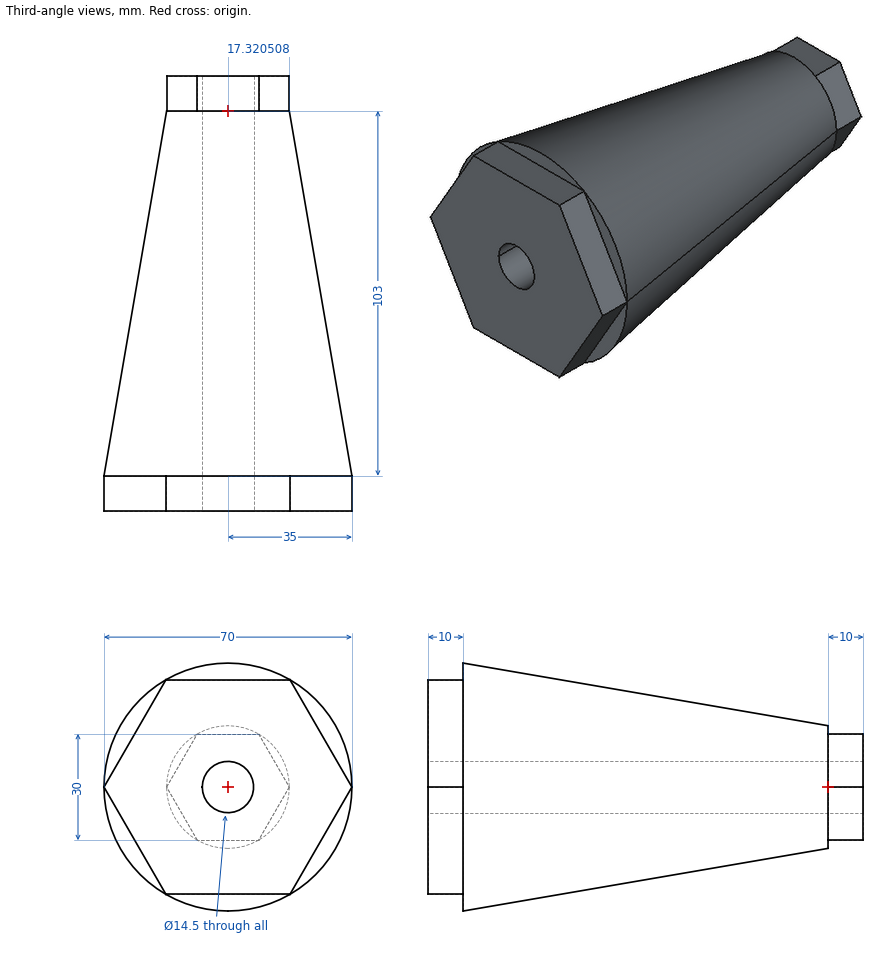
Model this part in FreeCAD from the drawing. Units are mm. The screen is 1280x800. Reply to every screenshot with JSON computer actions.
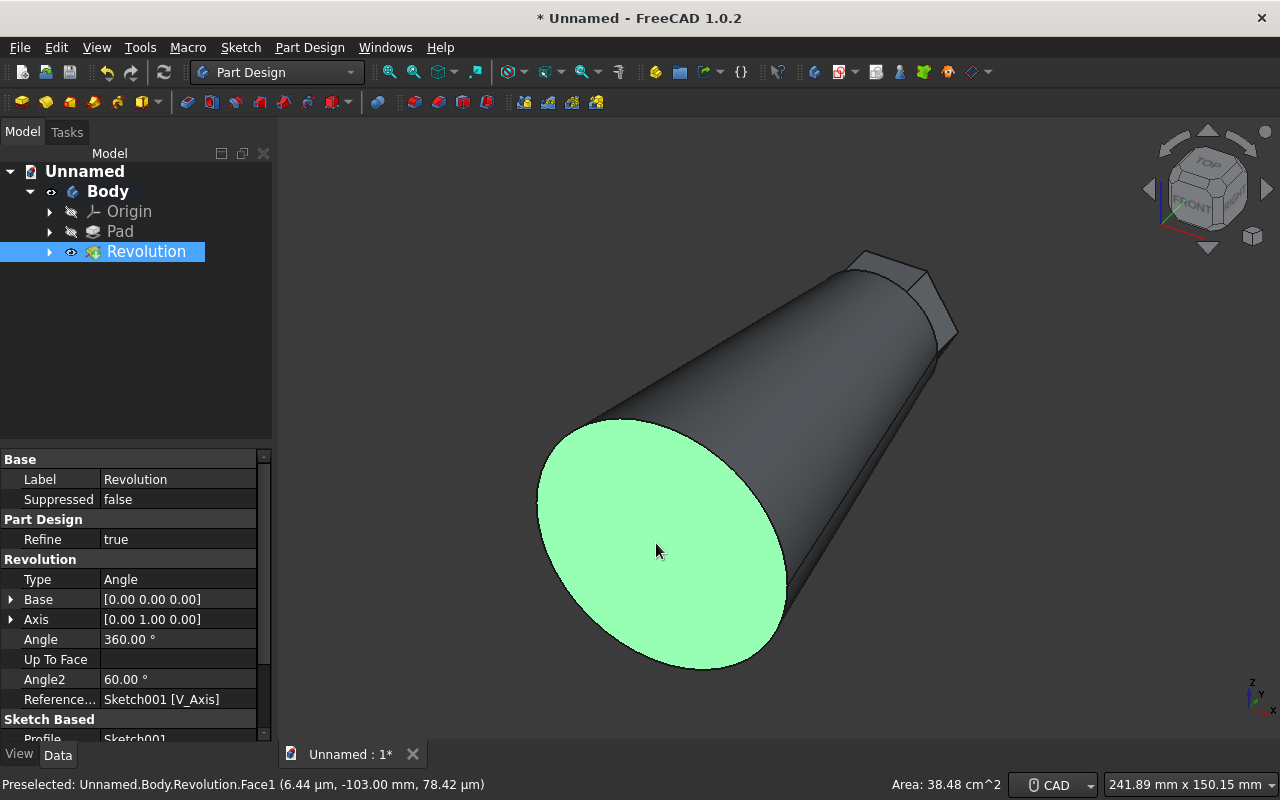
{"action": "left_click", "coordinate": [840, 72]}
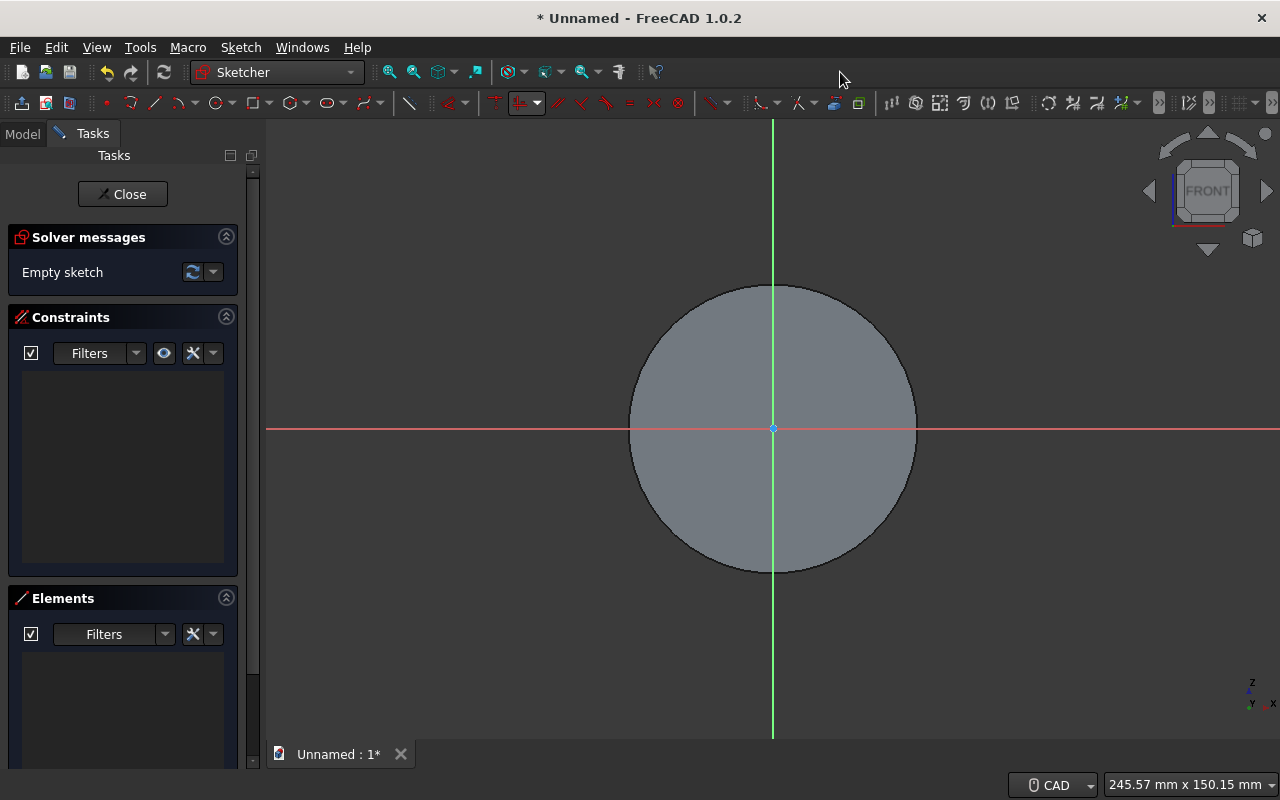
{"action": "scroll", "coordinate": [912, 429], "scroll_direction": "up", "scroll_amount": 2}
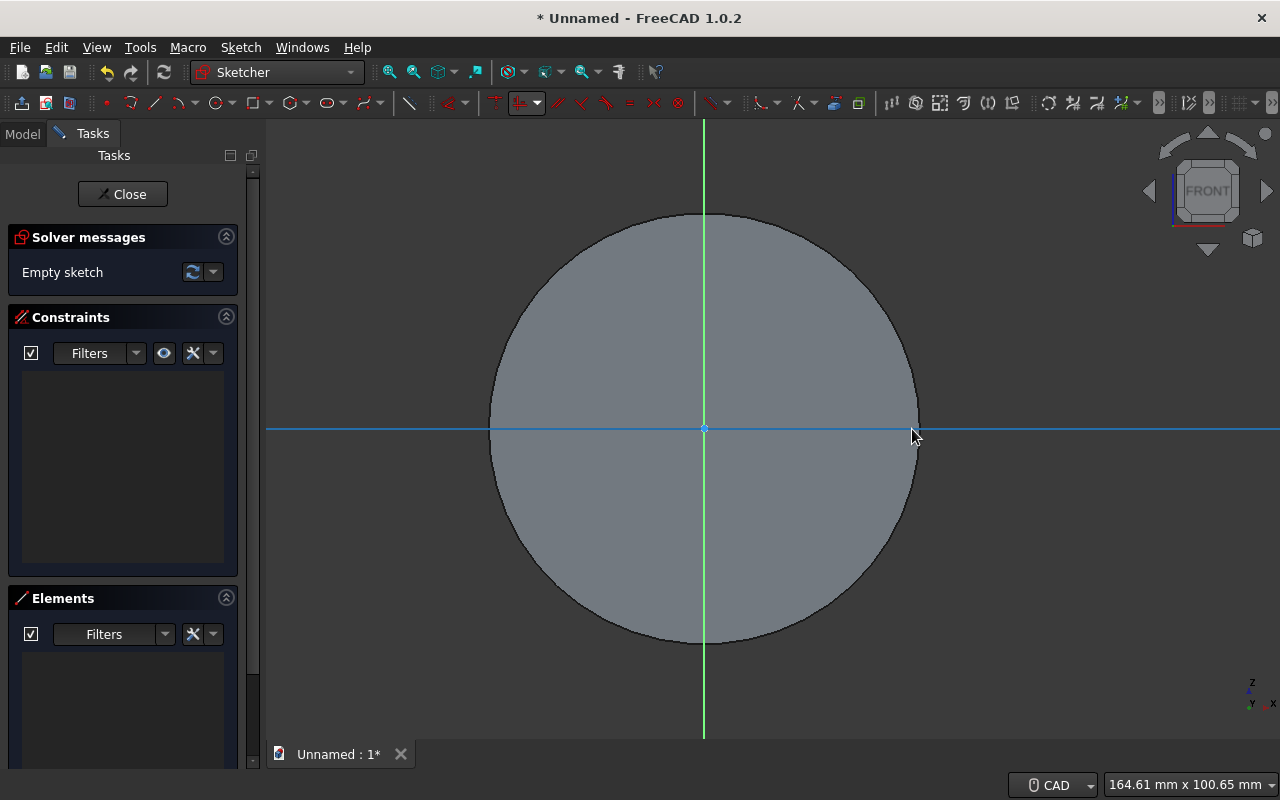
{"action": "left_click", "coordinate": [290, 104]}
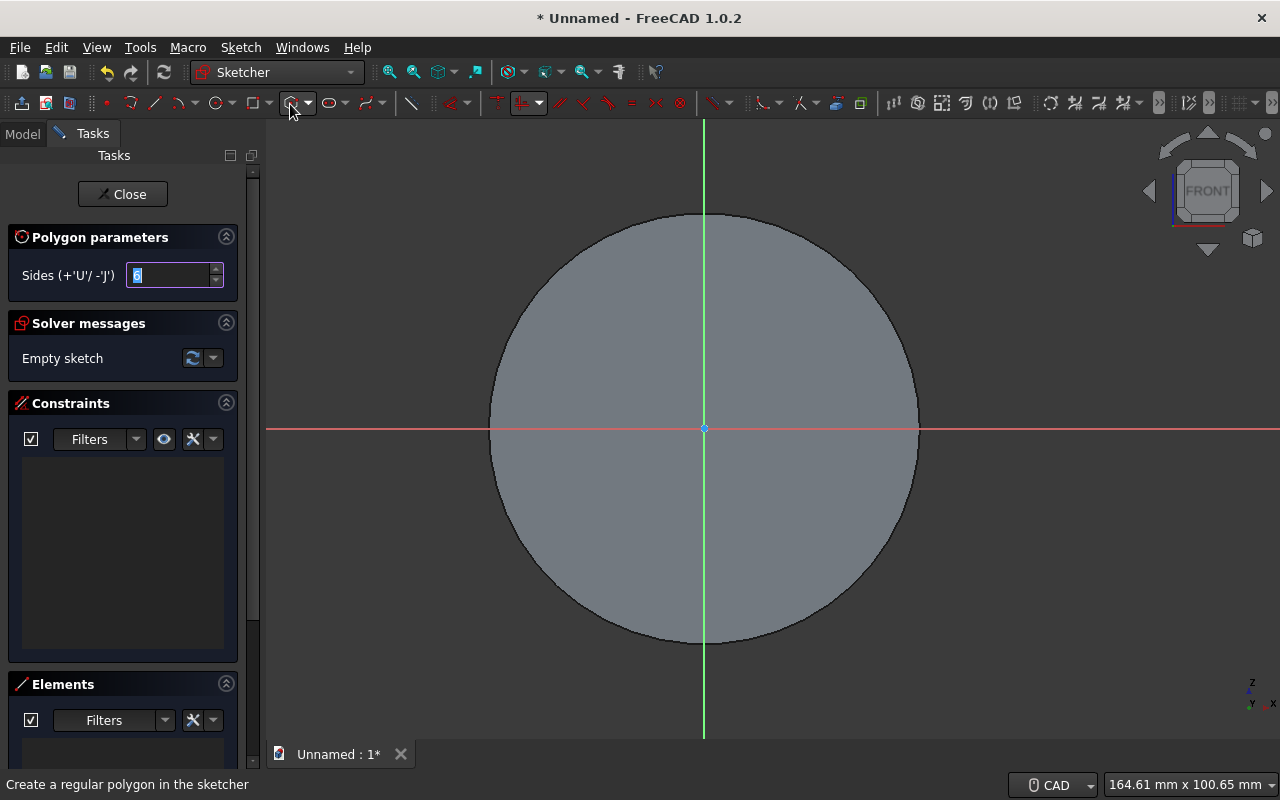
{"action": "left_click", "coordinate": [704, 429]}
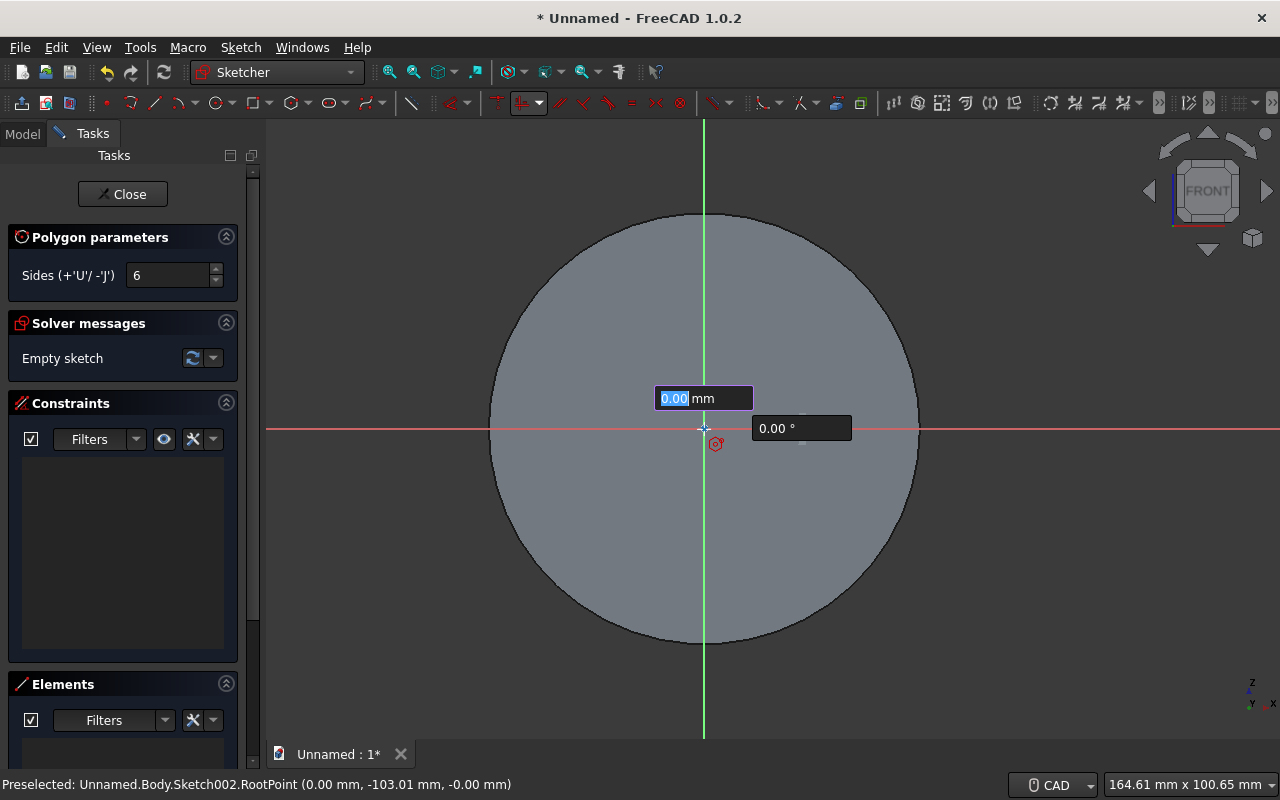
{"action": "left_click", "coordinate": [489, 429]}
{"action": "right_click", "coordinate": [489, 429]}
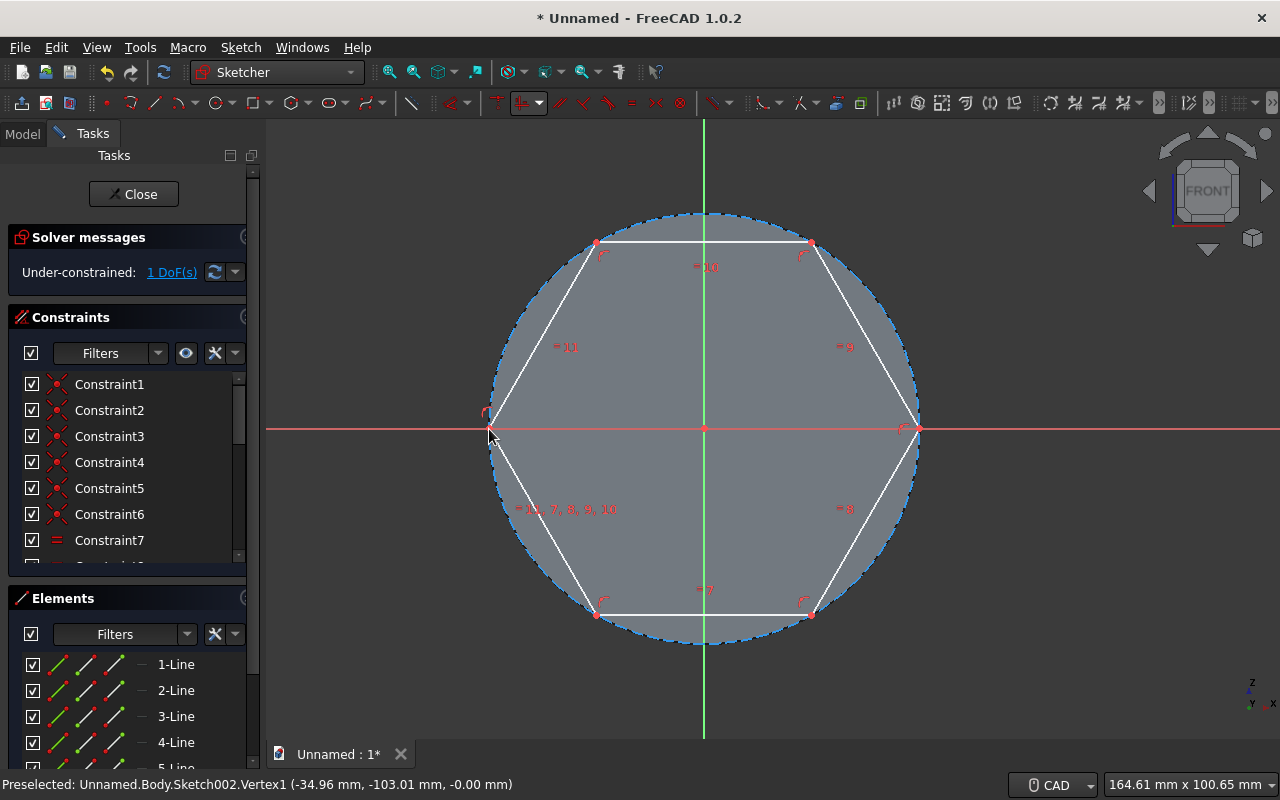
{"action": "left_click", "coordinate": [450, 104]}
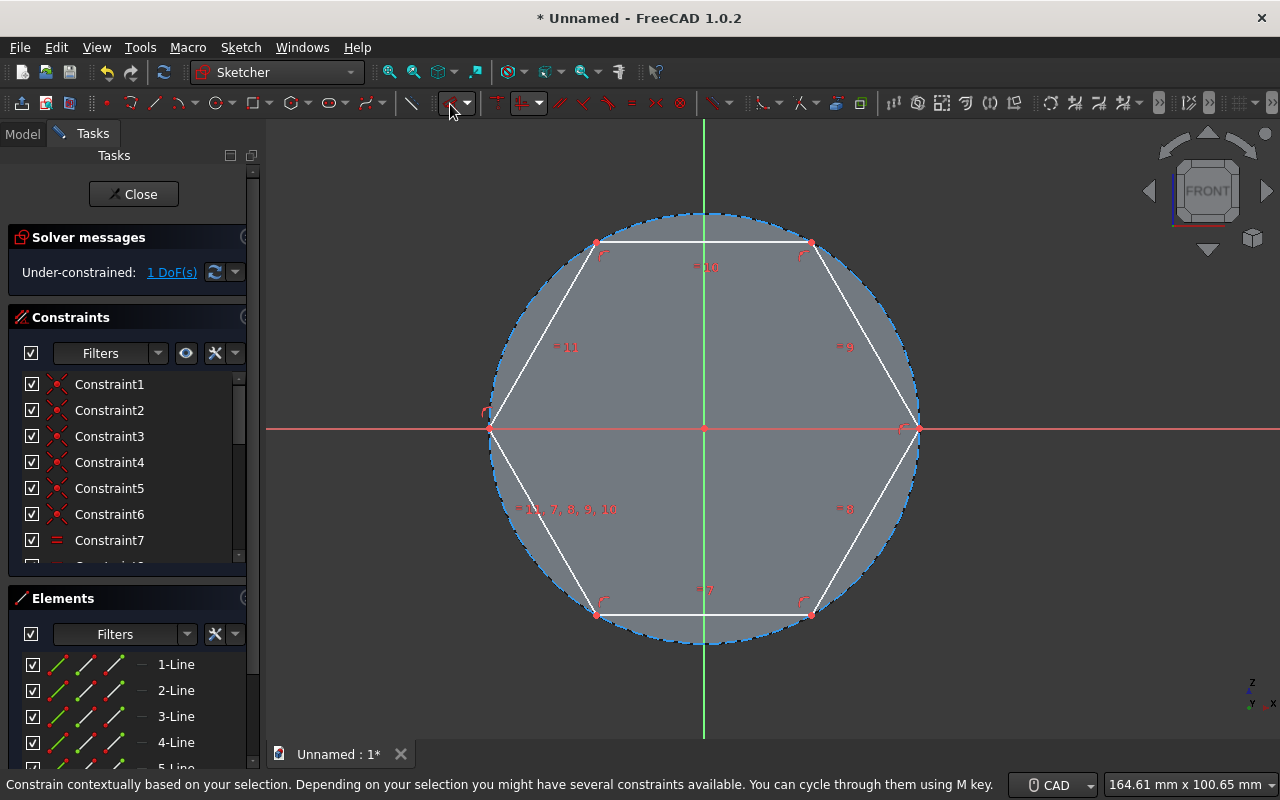
{"action": "left_click", "coordinate": [489, 429]}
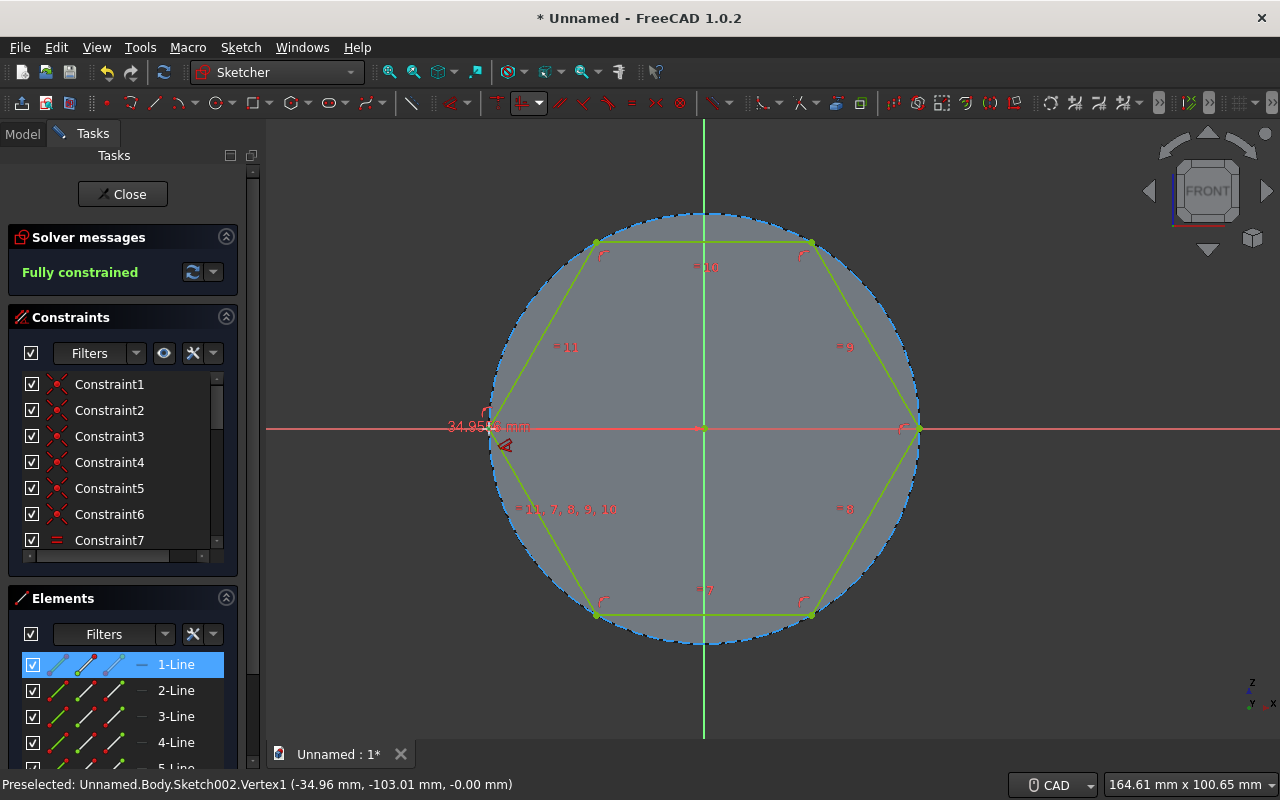
{"action": "left_click", "coordinate": [920, 429]}
{"action": "left_click", "coordinate": [605, 463]}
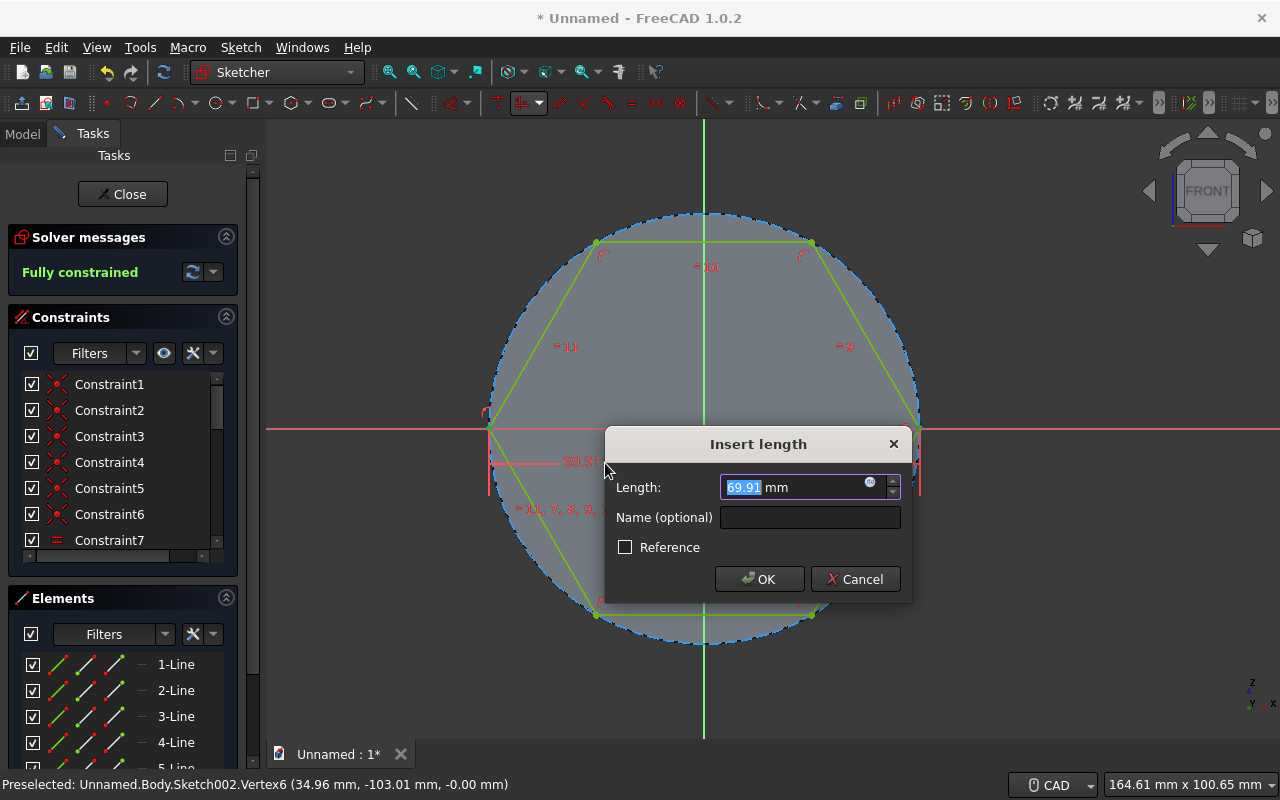
{"action": "type", "text": "70"}
{"action": "key", "text": "Return"}
{"action": "key", "text": "Escape"}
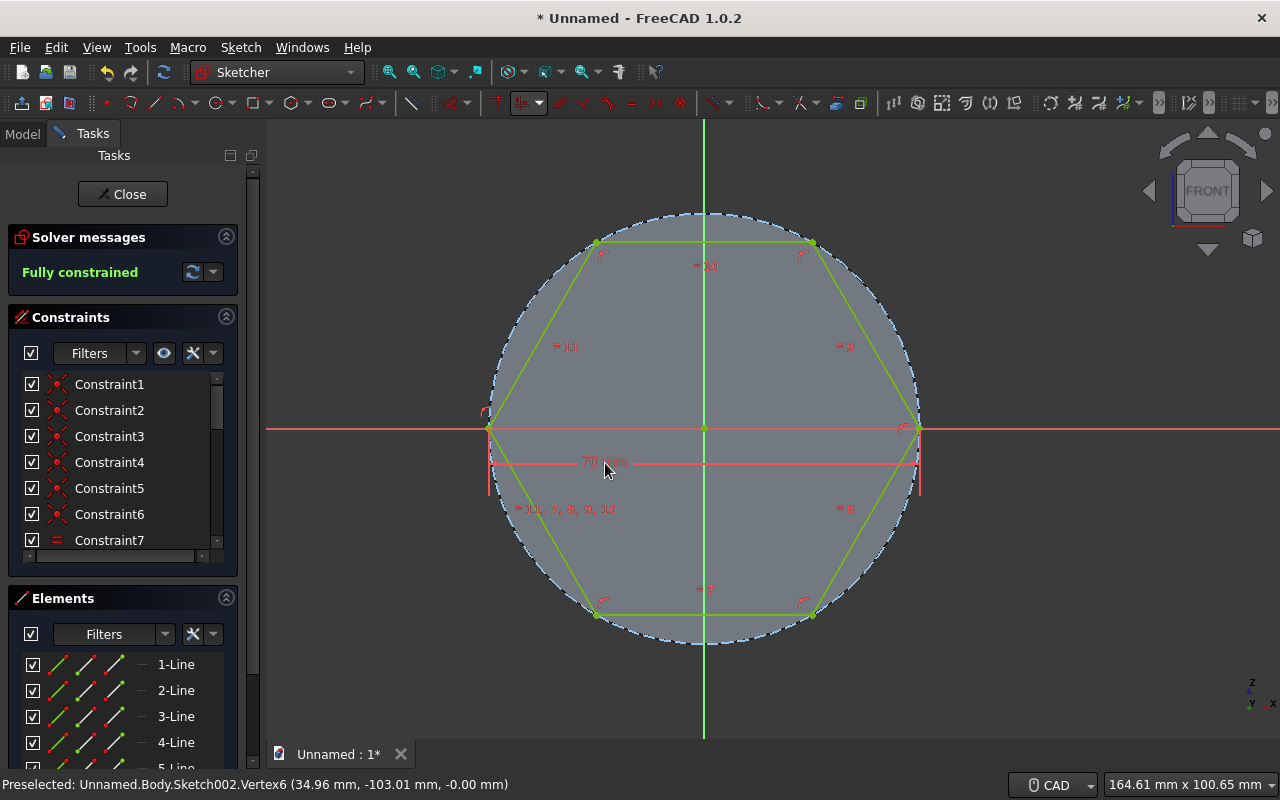
{"action": "left_click", "coordinate": [123, 194]}